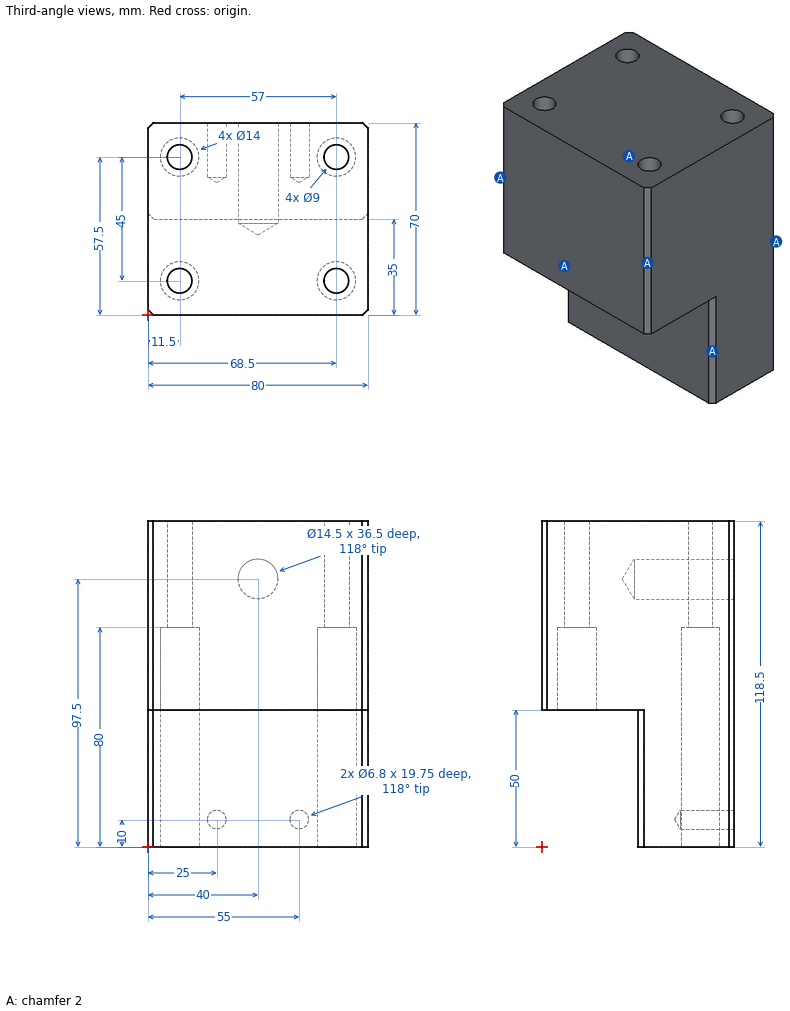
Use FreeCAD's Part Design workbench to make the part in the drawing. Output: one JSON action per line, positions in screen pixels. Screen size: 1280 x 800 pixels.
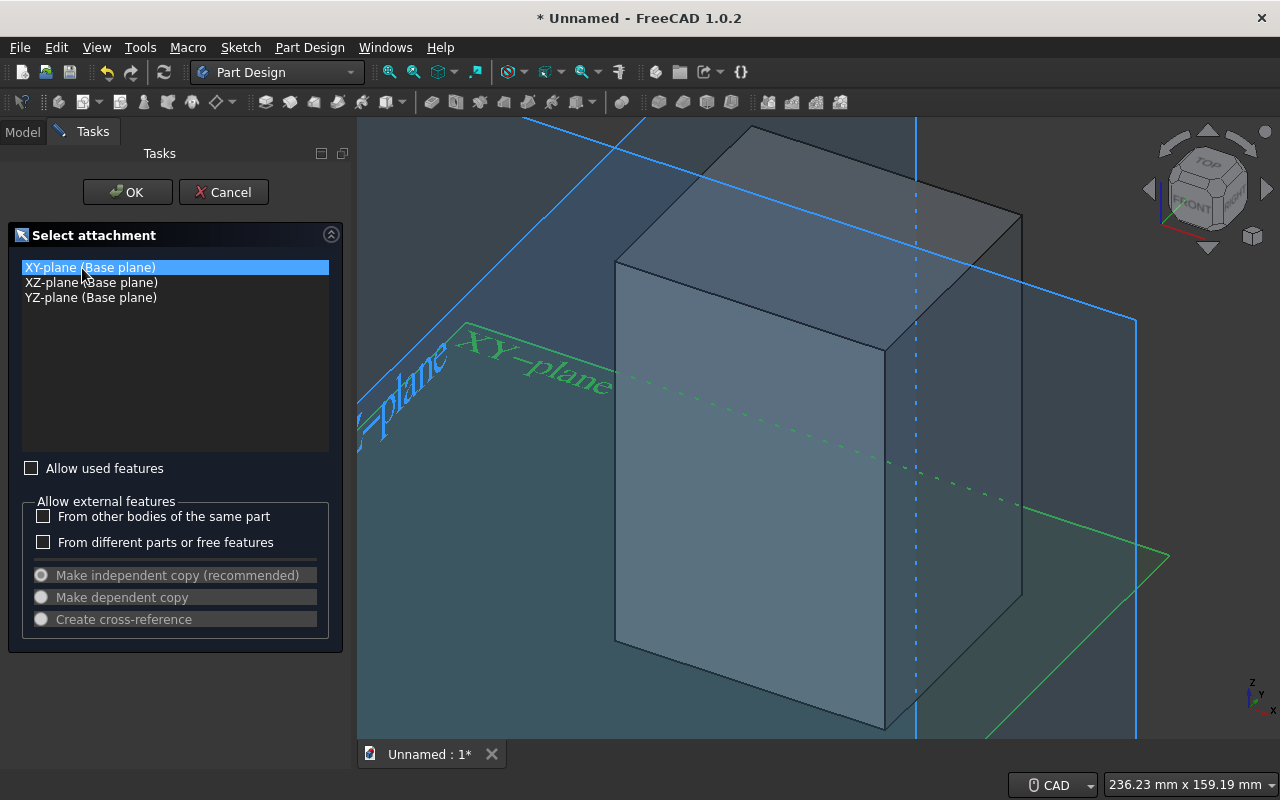
{"action": "left_click", "coordinate": [128, 192]}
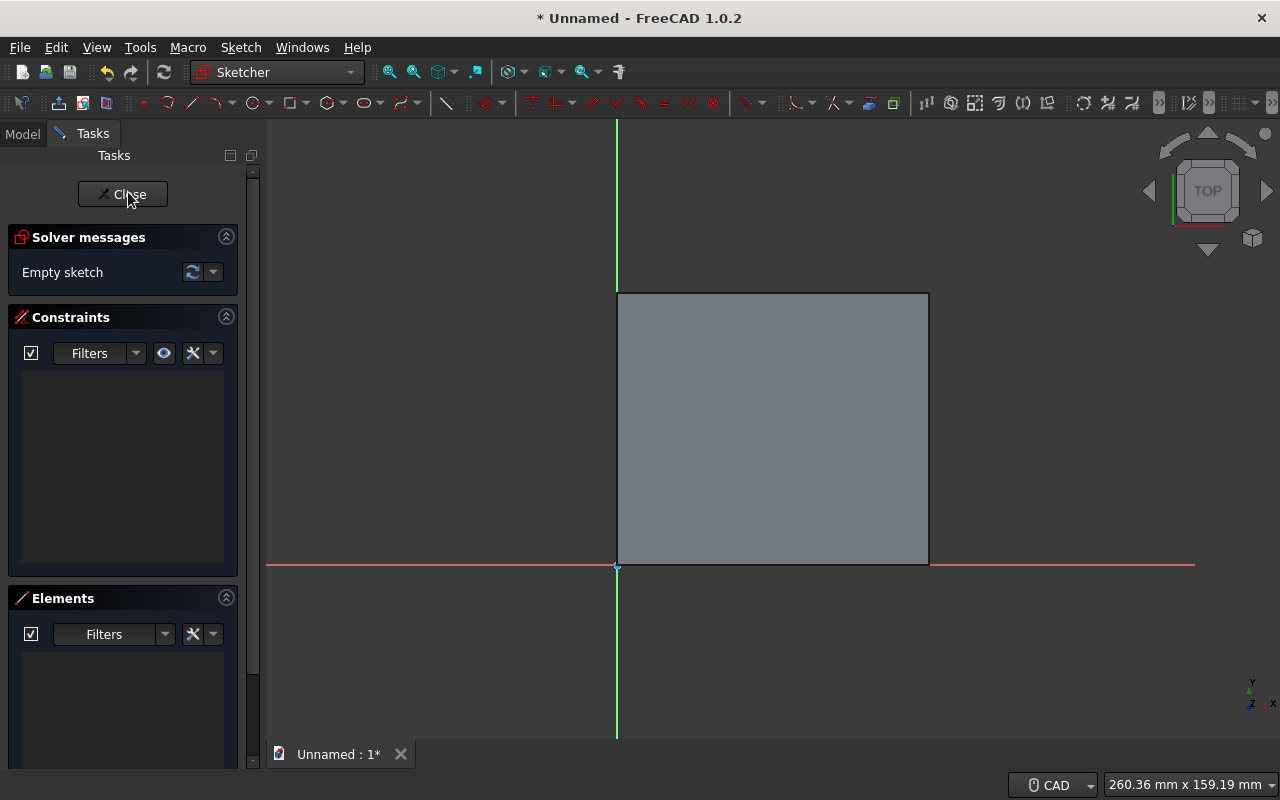
{"action": "key", "text": "q s"}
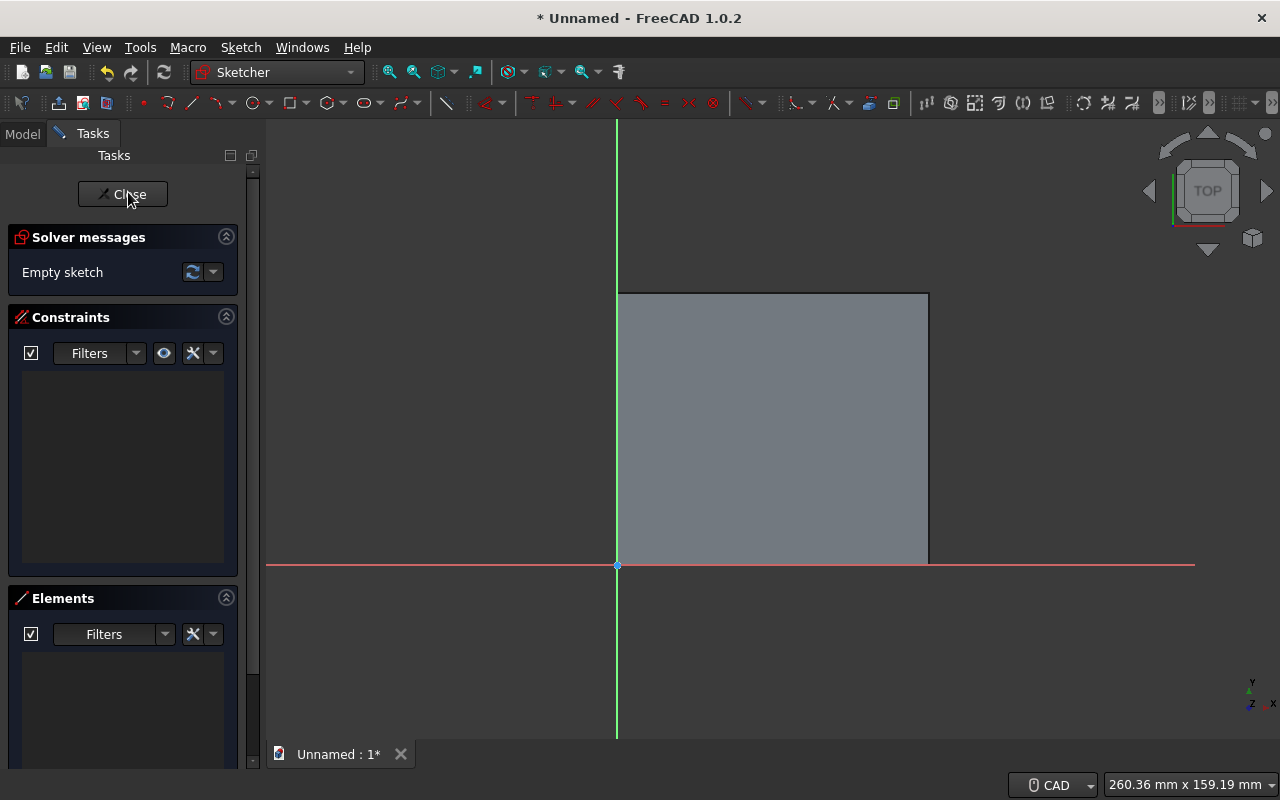
{"action": "scroll", "coordinate": [886, 461], "scroll_direction": "up", "scroll_amount": 2}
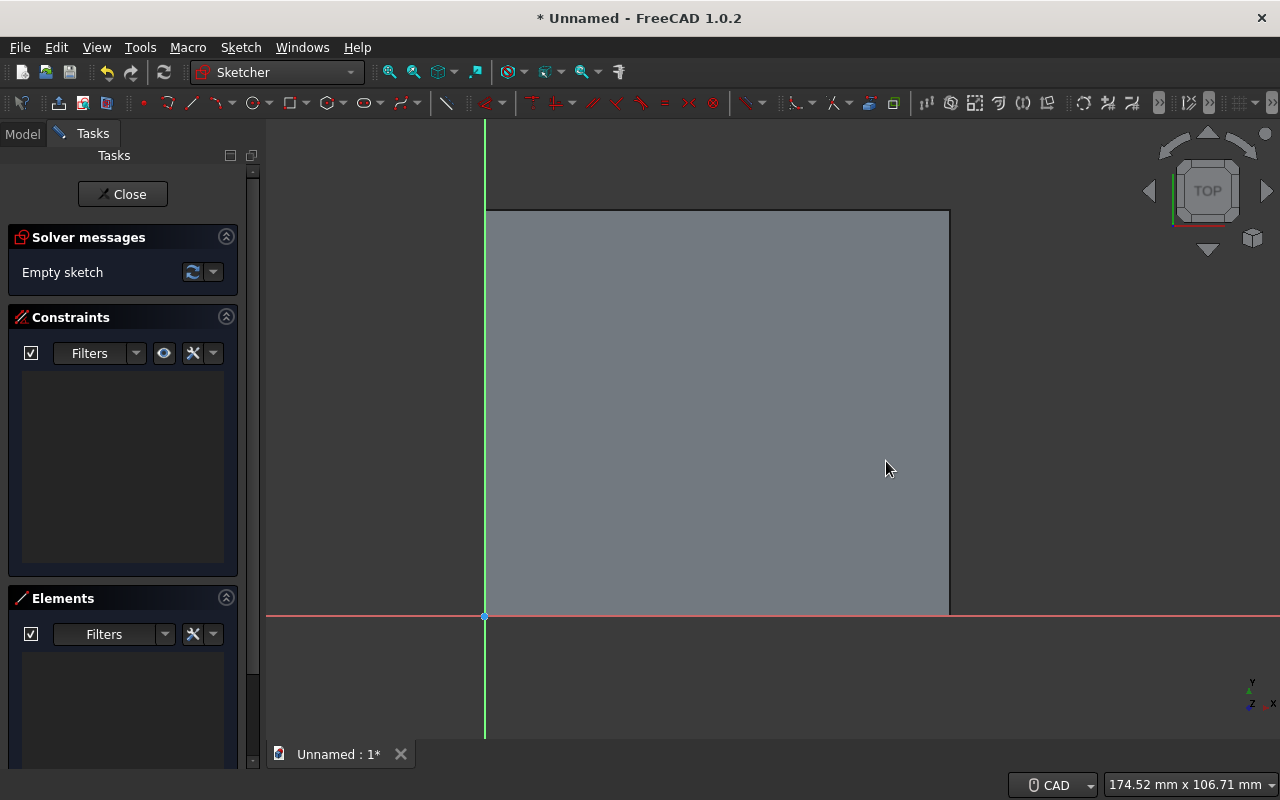
{"action": "key", "text": "g c"}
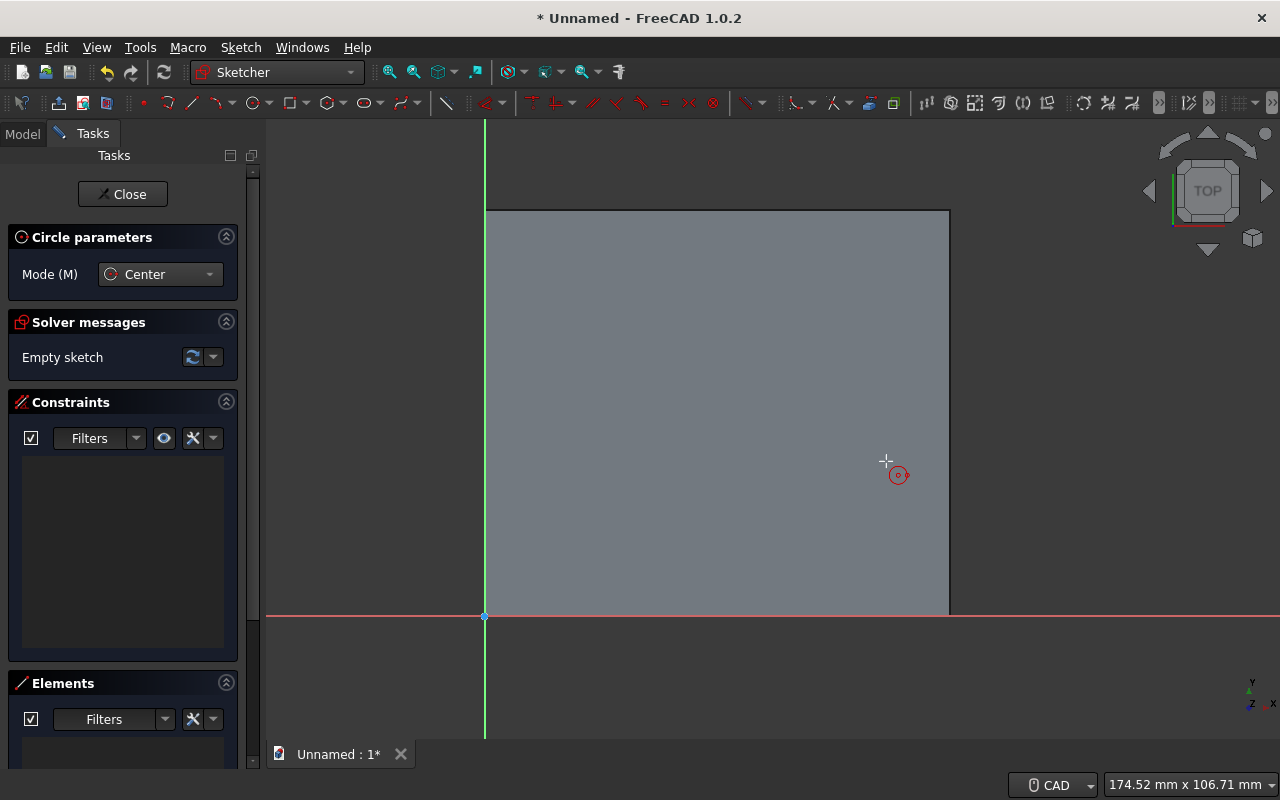
{"action": "left_click", "coordinate": [552, 282]}
{"action": "left_click", "coordinate": [580, 254]}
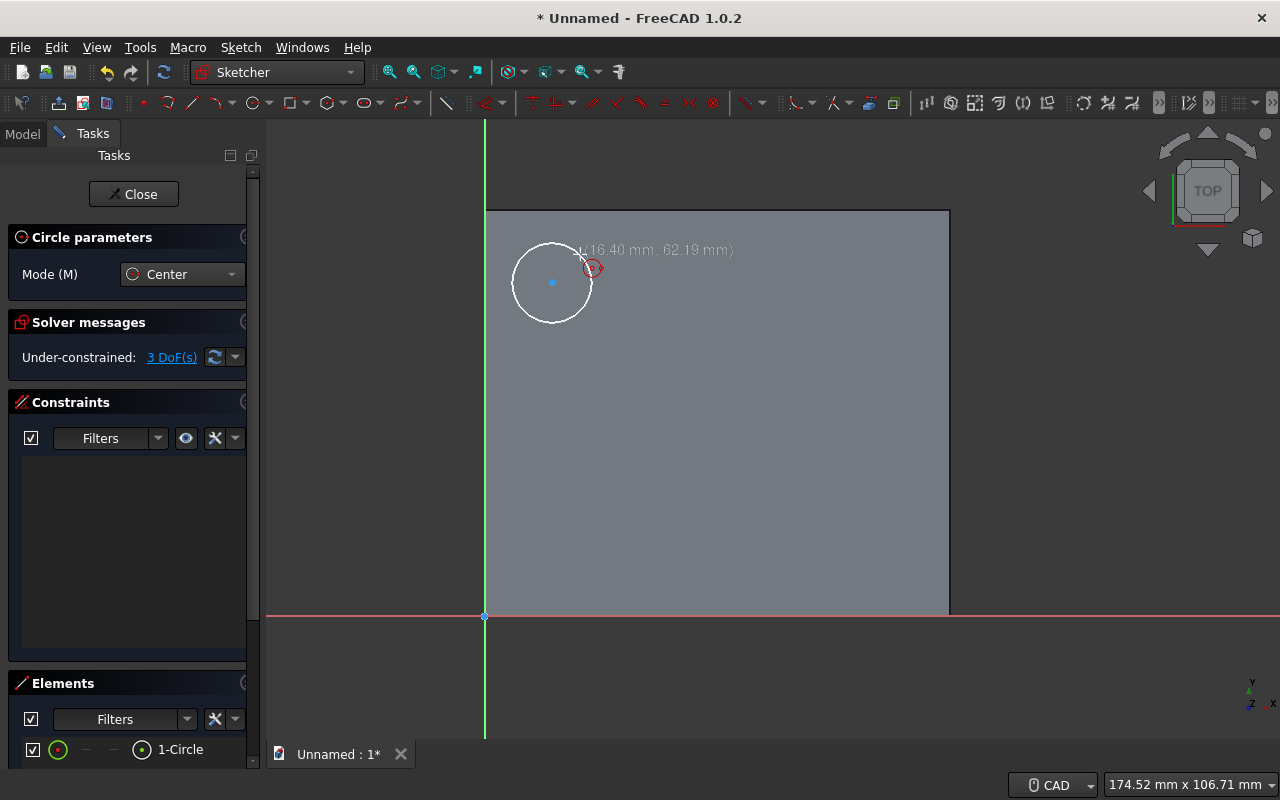
{"action": "left_click", "coordinate": [552, 544]}
{"action": "left_click", "coordinate": [580, 515]}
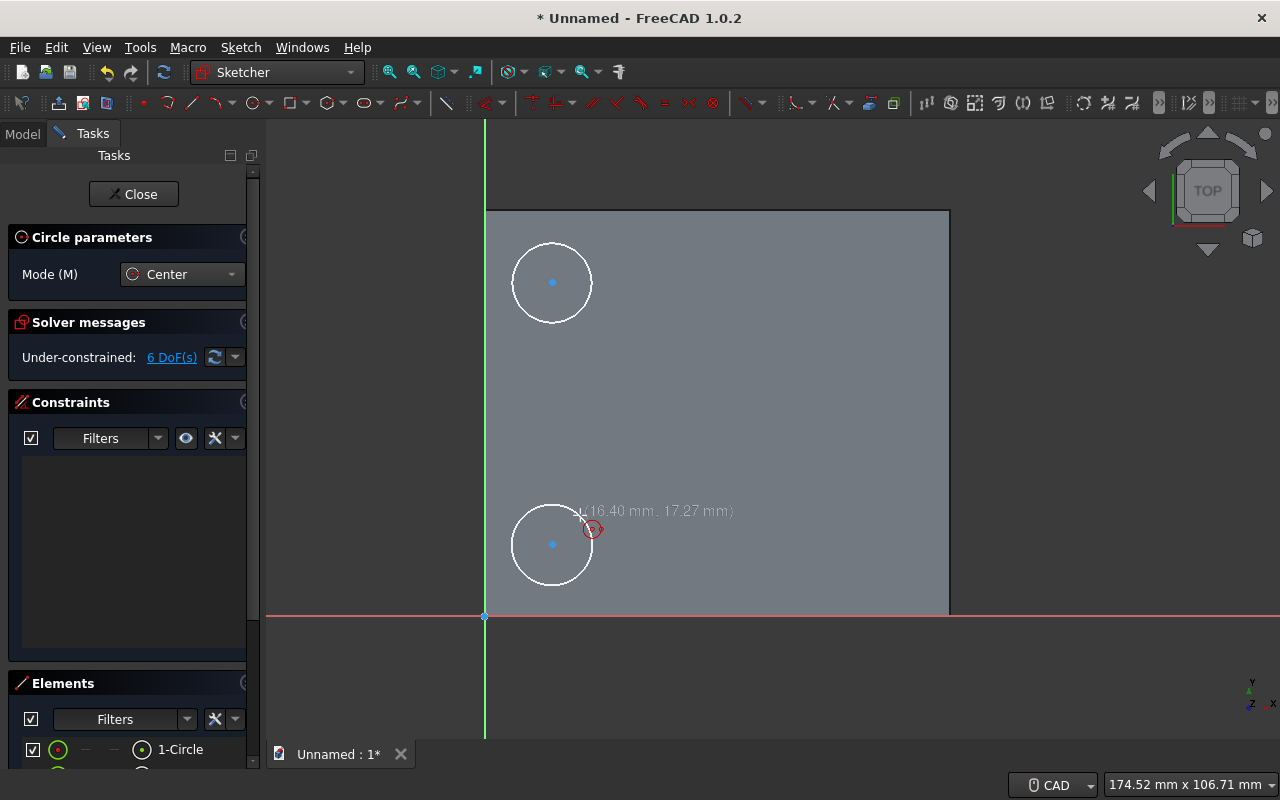
{"action": "left_click", "coordinate": [883, 282]}
{"action": "left_click", "coordinate": [911, 254]}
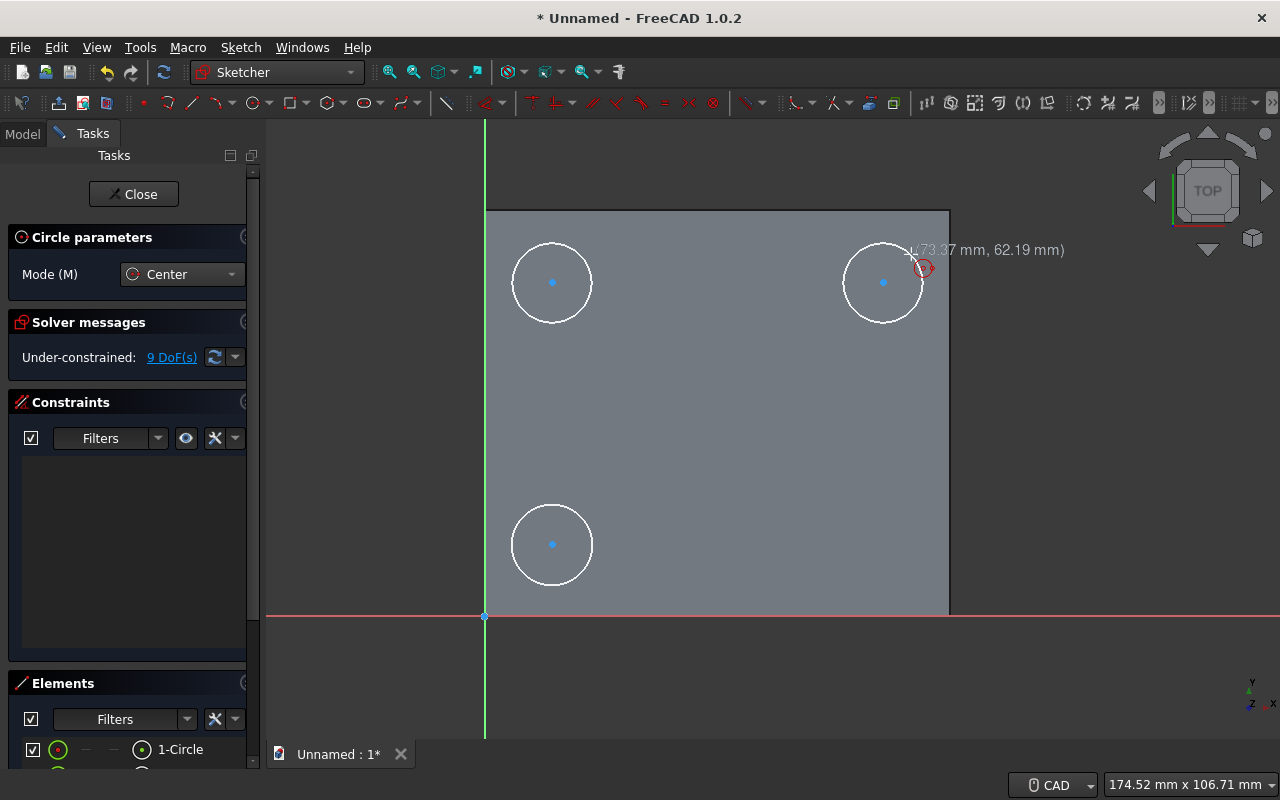
{"action": "left_click", "coordinate": [883, 544]}
{"action": "left_click", "coordinate": [911, 515]}
{"action": "key", "text": "Escape"}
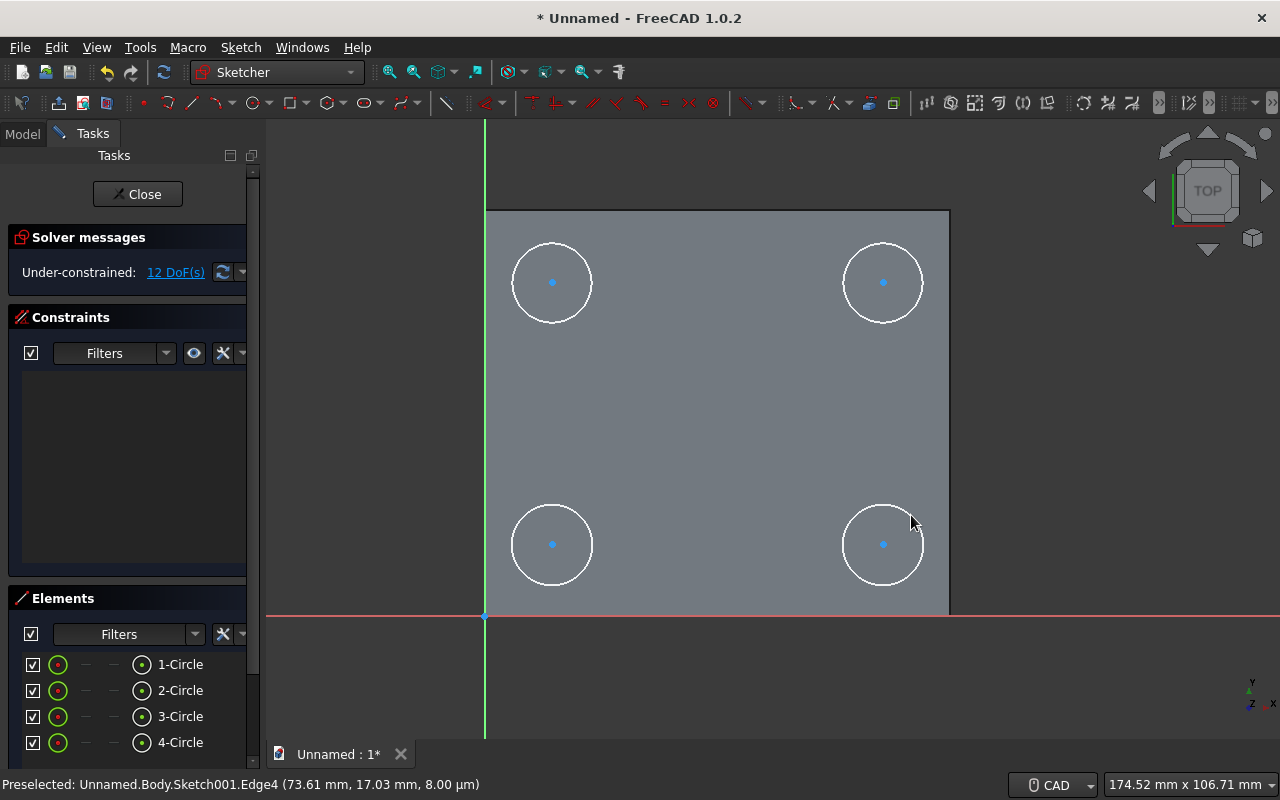
{"action": "left_click", "coordinate": [580, 255]}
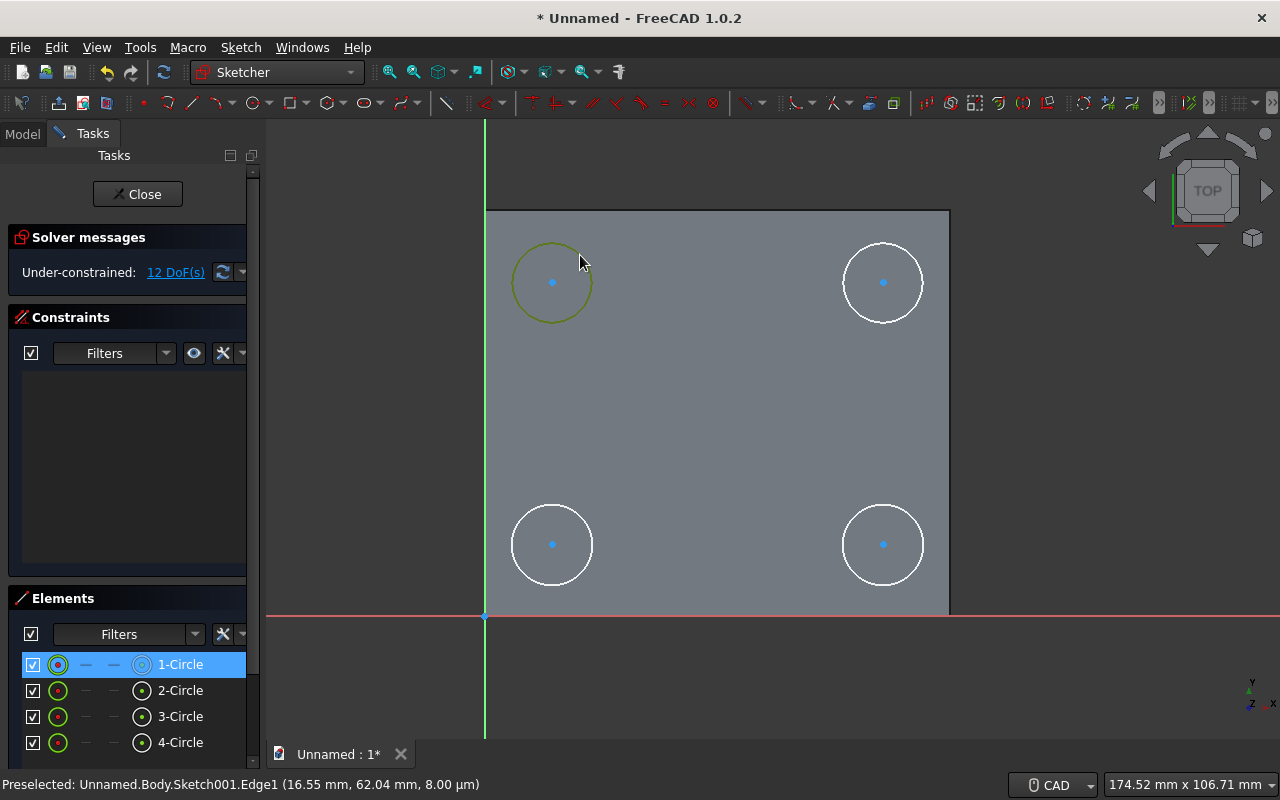
{"action": "left_click", "coordinate": [580, 516]}